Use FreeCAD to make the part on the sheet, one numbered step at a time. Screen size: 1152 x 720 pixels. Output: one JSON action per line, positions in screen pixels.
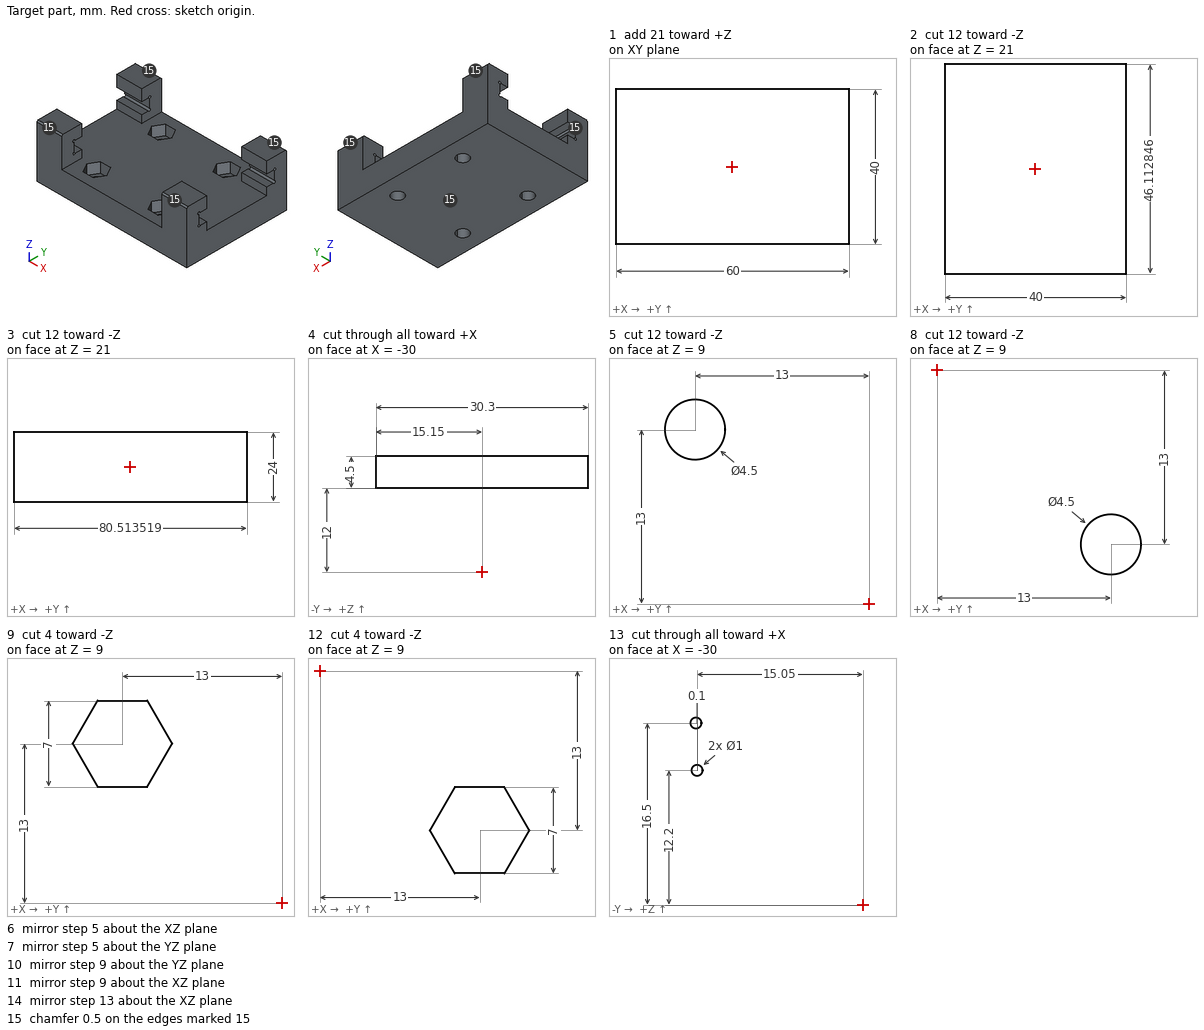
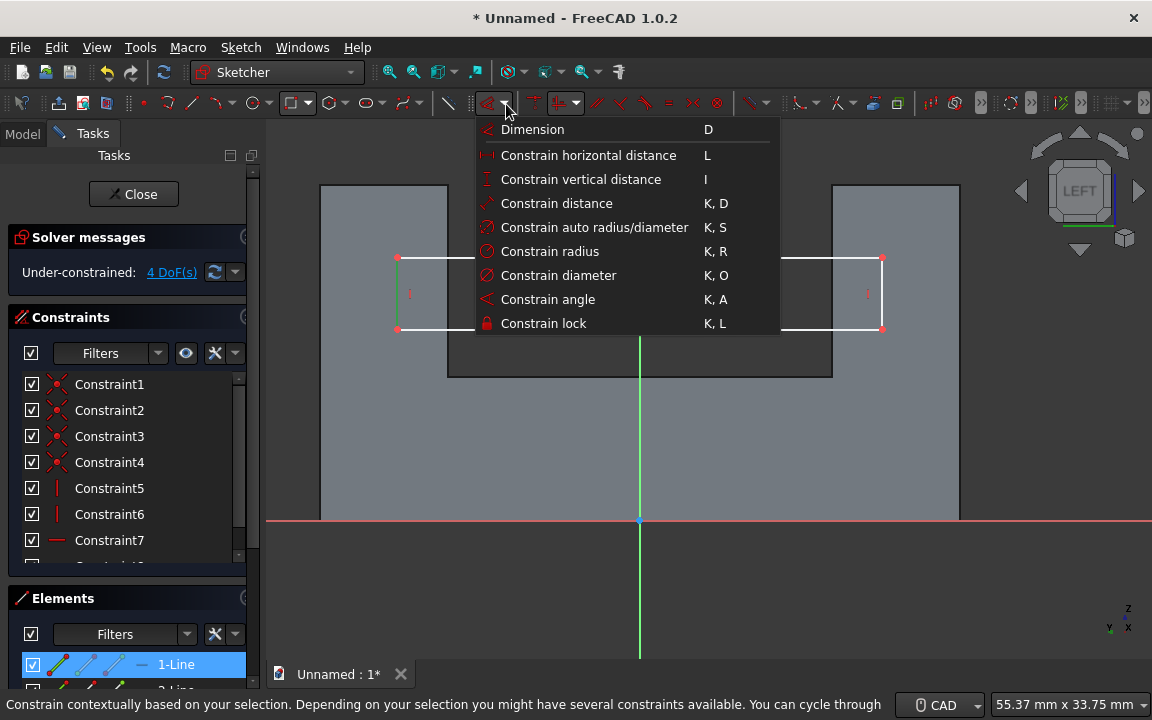
{"action": "left_click", "coordinate": [628, 179]}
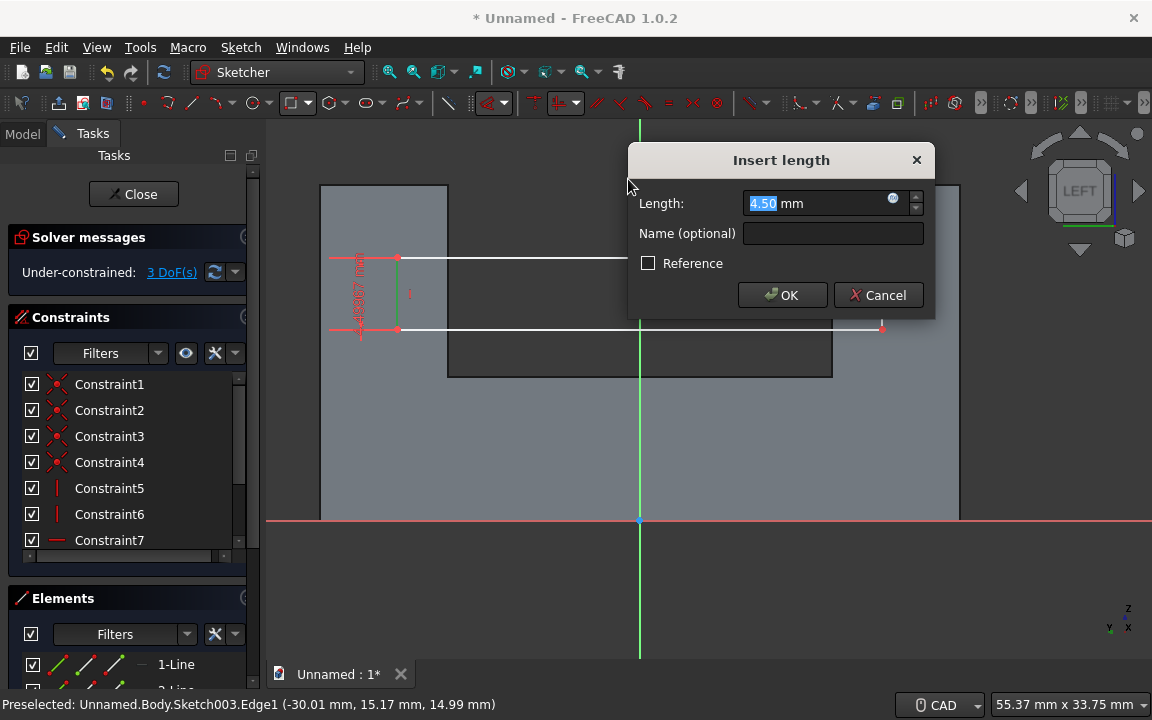
{"action": "type", "text": "4.5"}
{"action": "key", "text": "Return"}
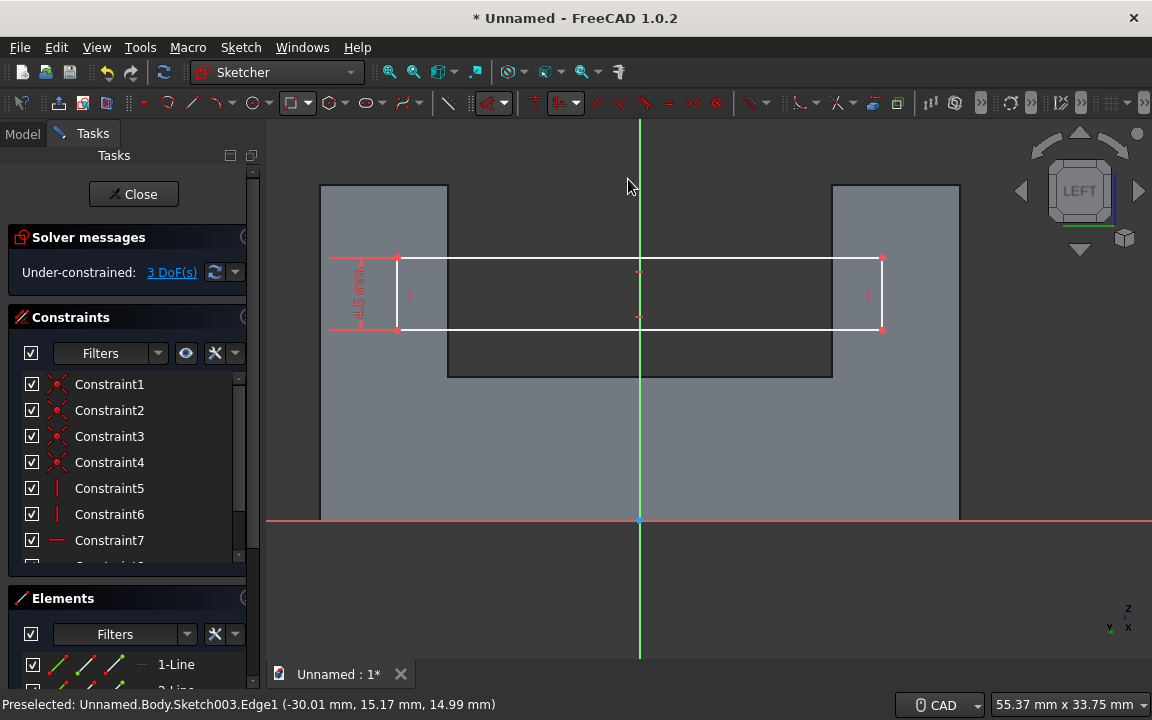
{"action": "left_click", "coordinate": [397, 330]}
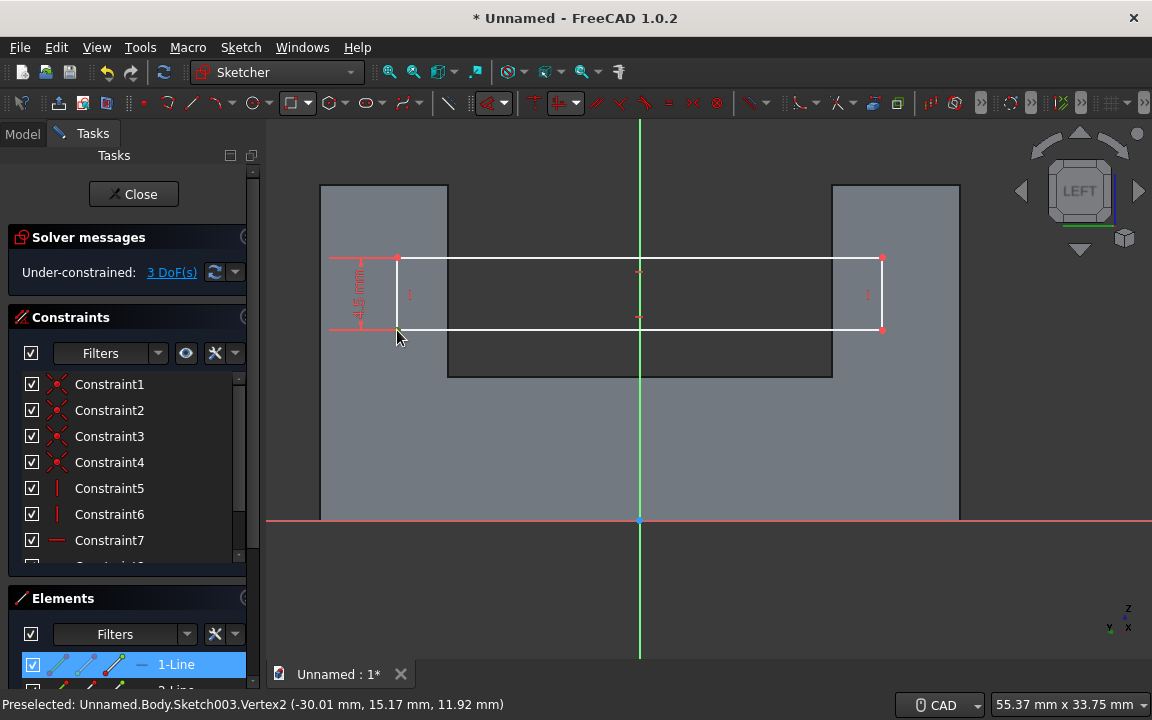
{"action": "left_click", "coordinate": [506, 104]}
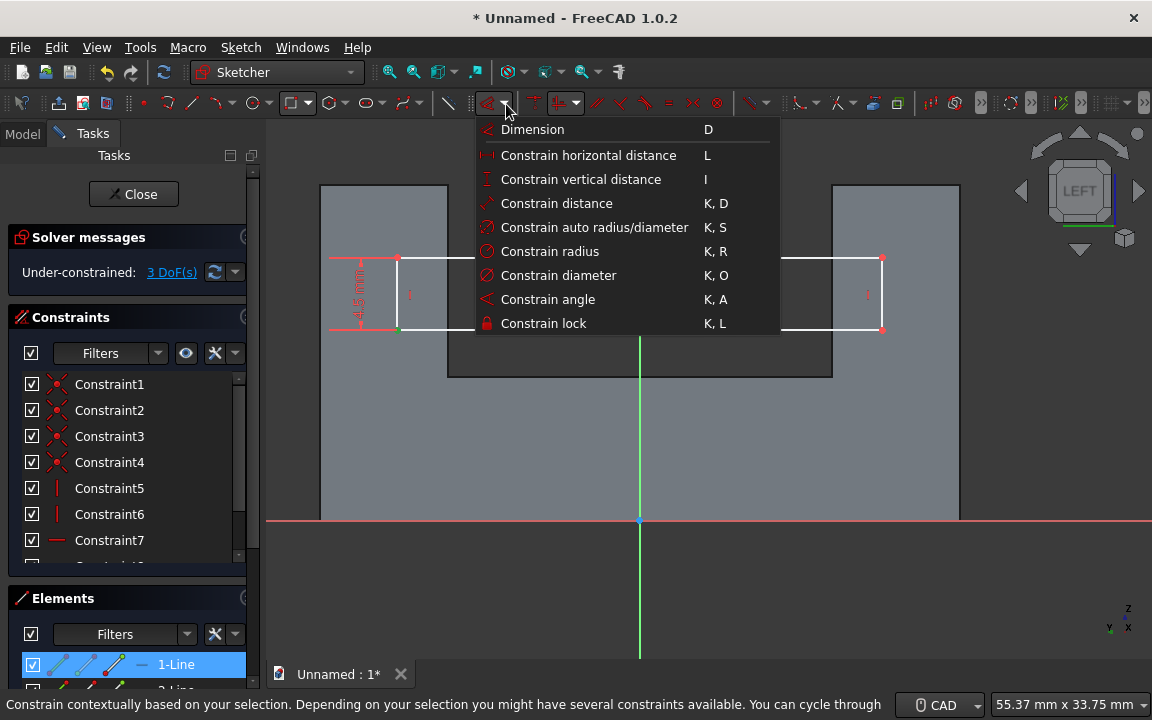
{"action": "left_click", "coordinate": [628, 179]}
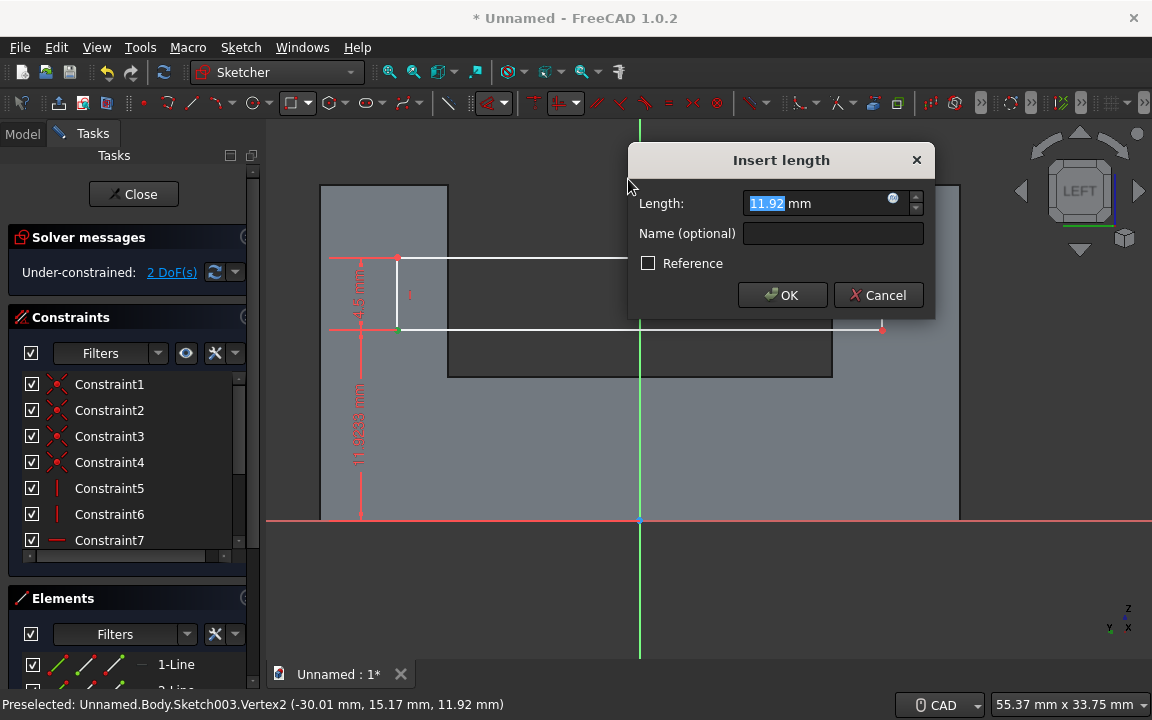
{"action": "type", "text": "12"}
{"action": "key", "text": "Return"}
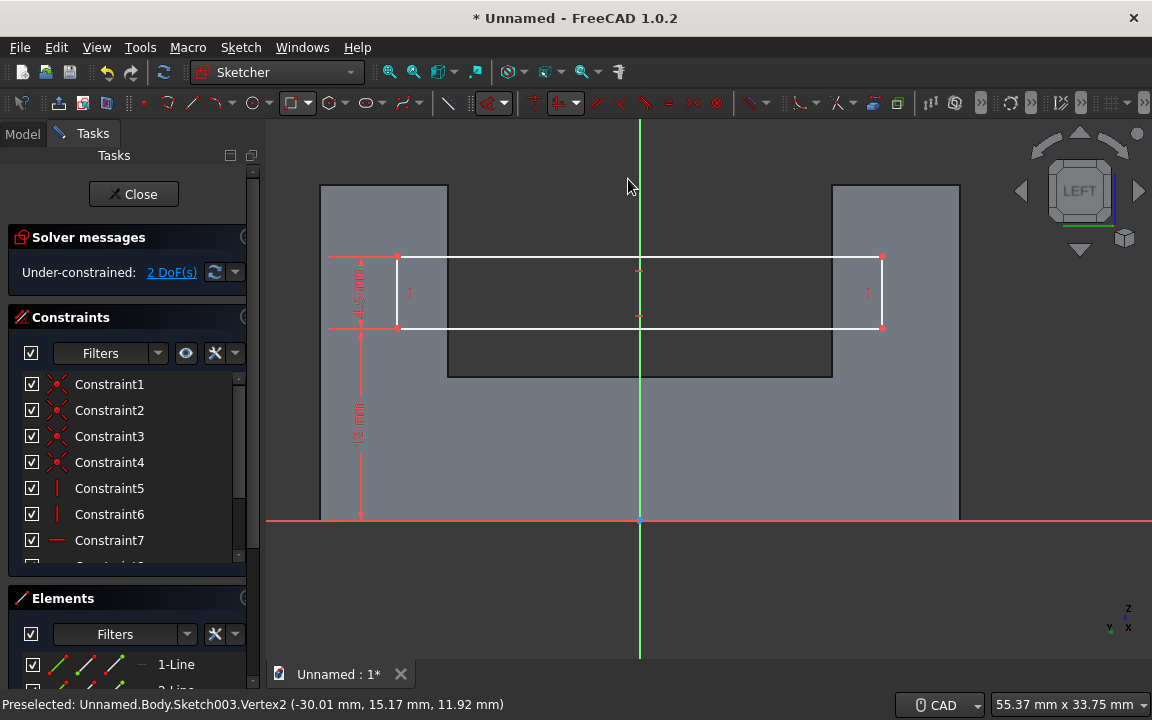
{"action": "left_click", "coordinate": [542, 329]}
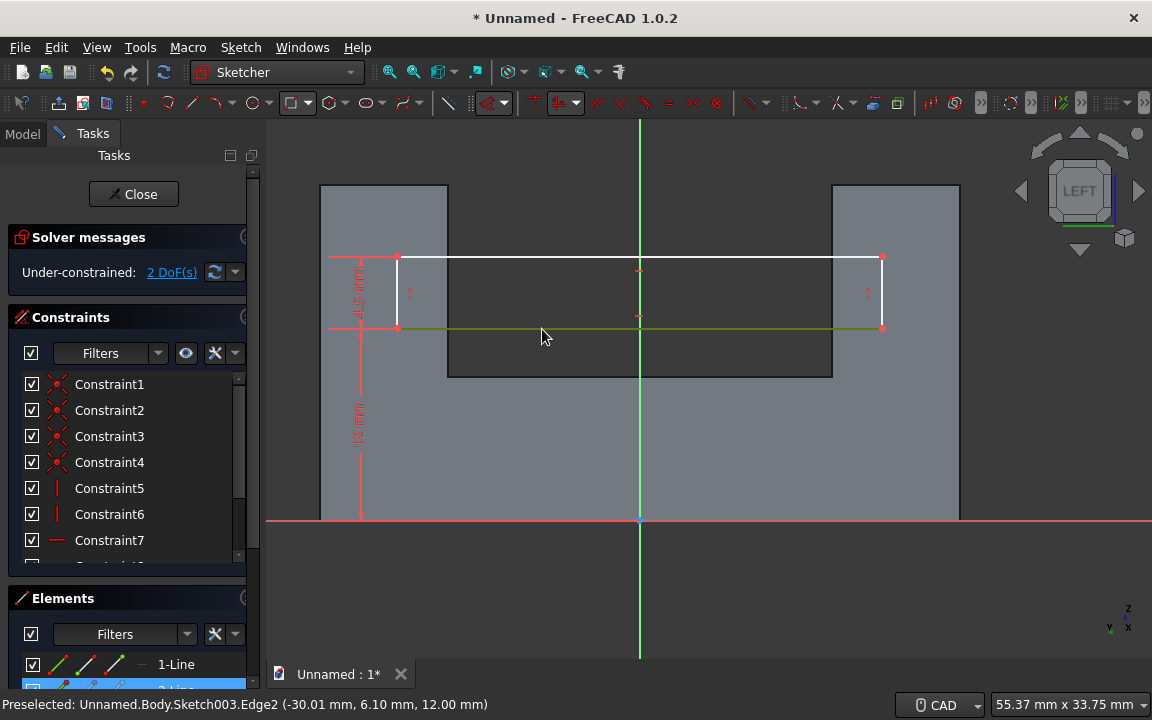
{"action": "left_click", "coordinate": [506, 104]}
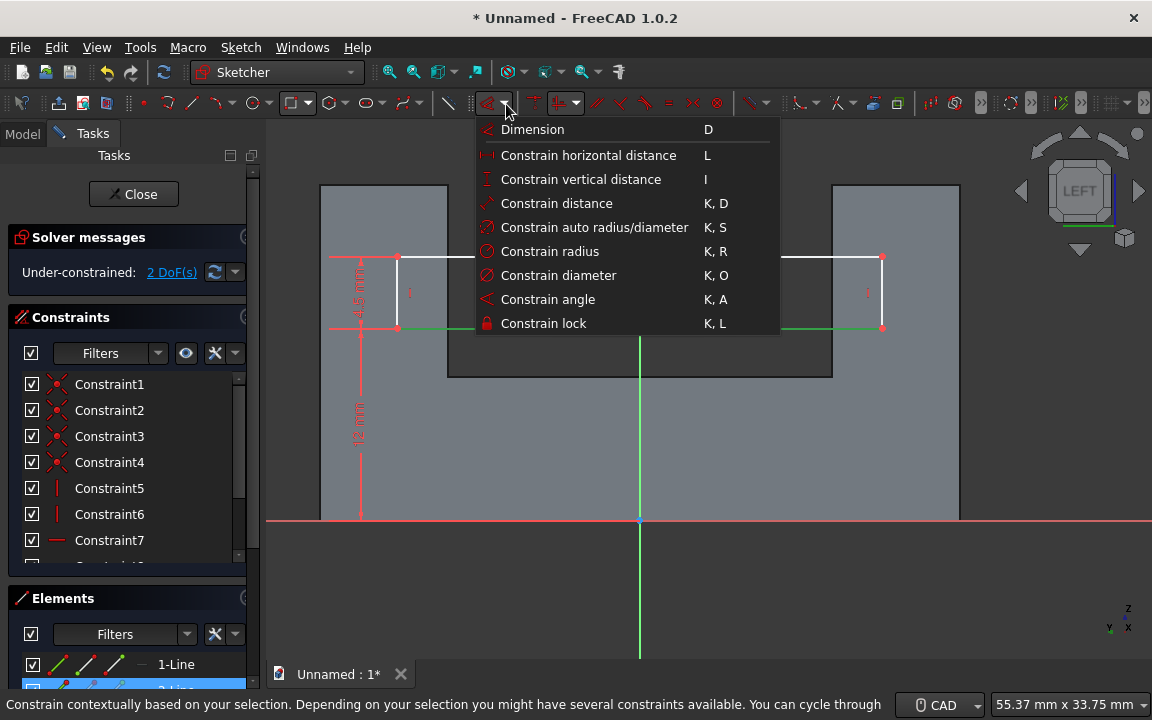
{"action": "left_click", "coordinate": [628, 155]}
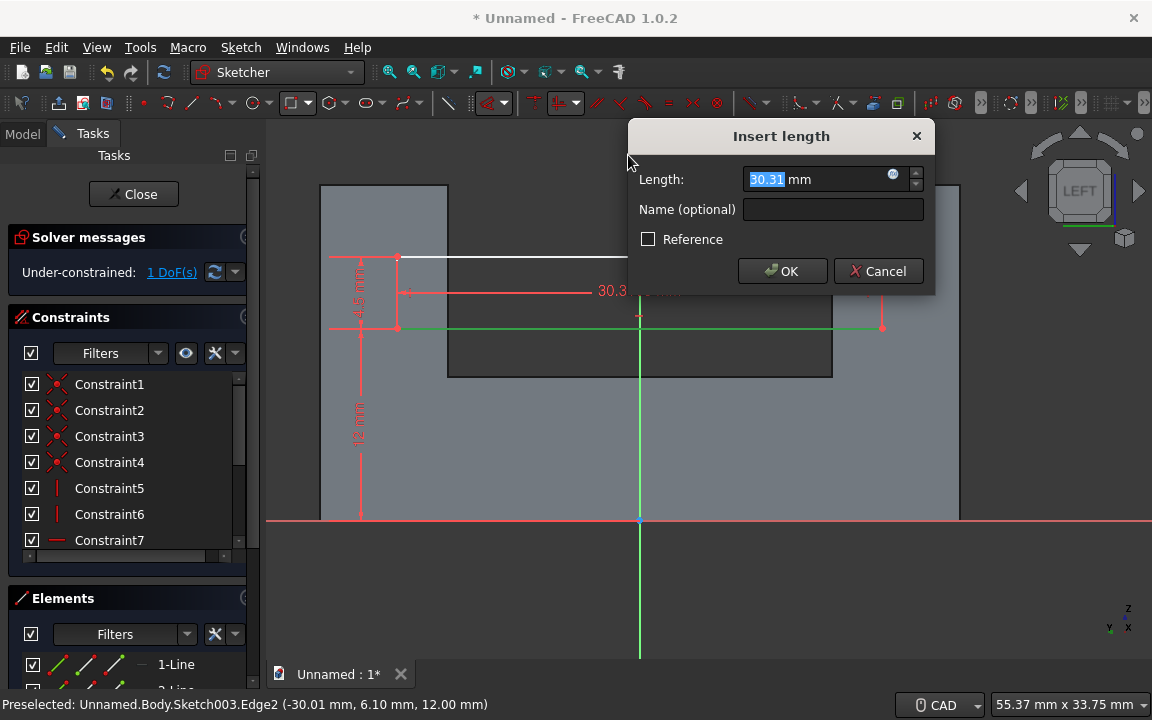
{"action": "type", "text": "30.3"}
{"action": "key", "text": "Return"}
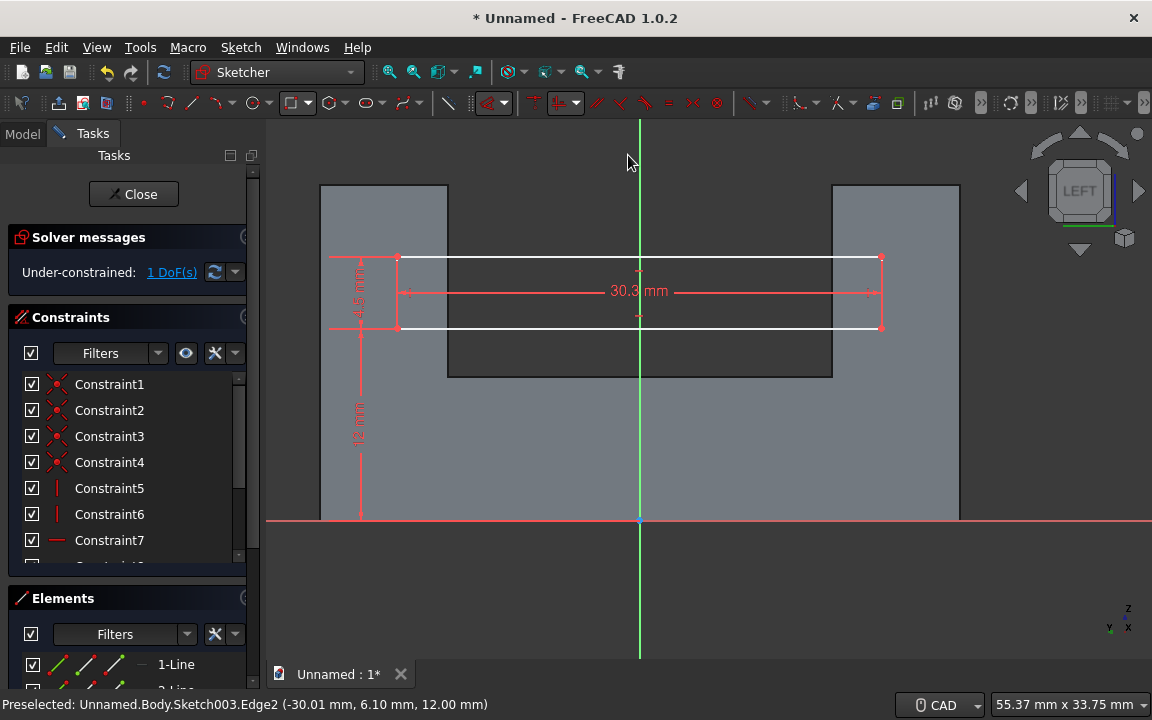
{"action": "left_click", "coordinate": [397, 257]}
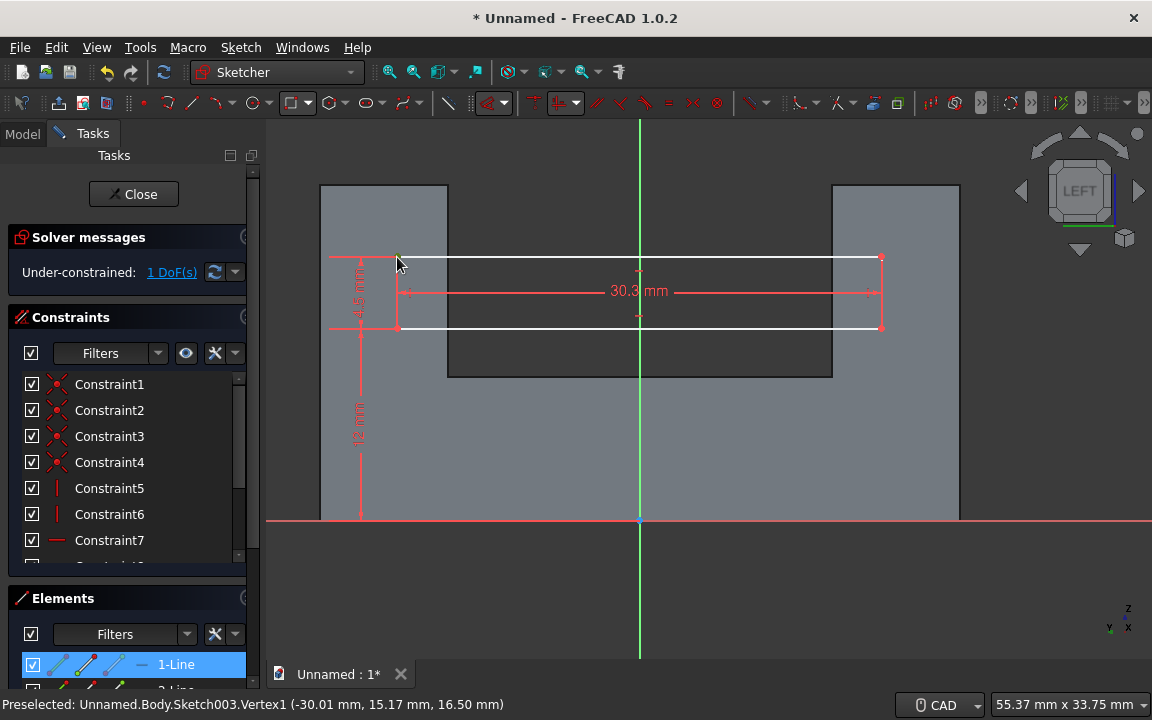
{"action": "left_click", "coordinate": [506, 104]}